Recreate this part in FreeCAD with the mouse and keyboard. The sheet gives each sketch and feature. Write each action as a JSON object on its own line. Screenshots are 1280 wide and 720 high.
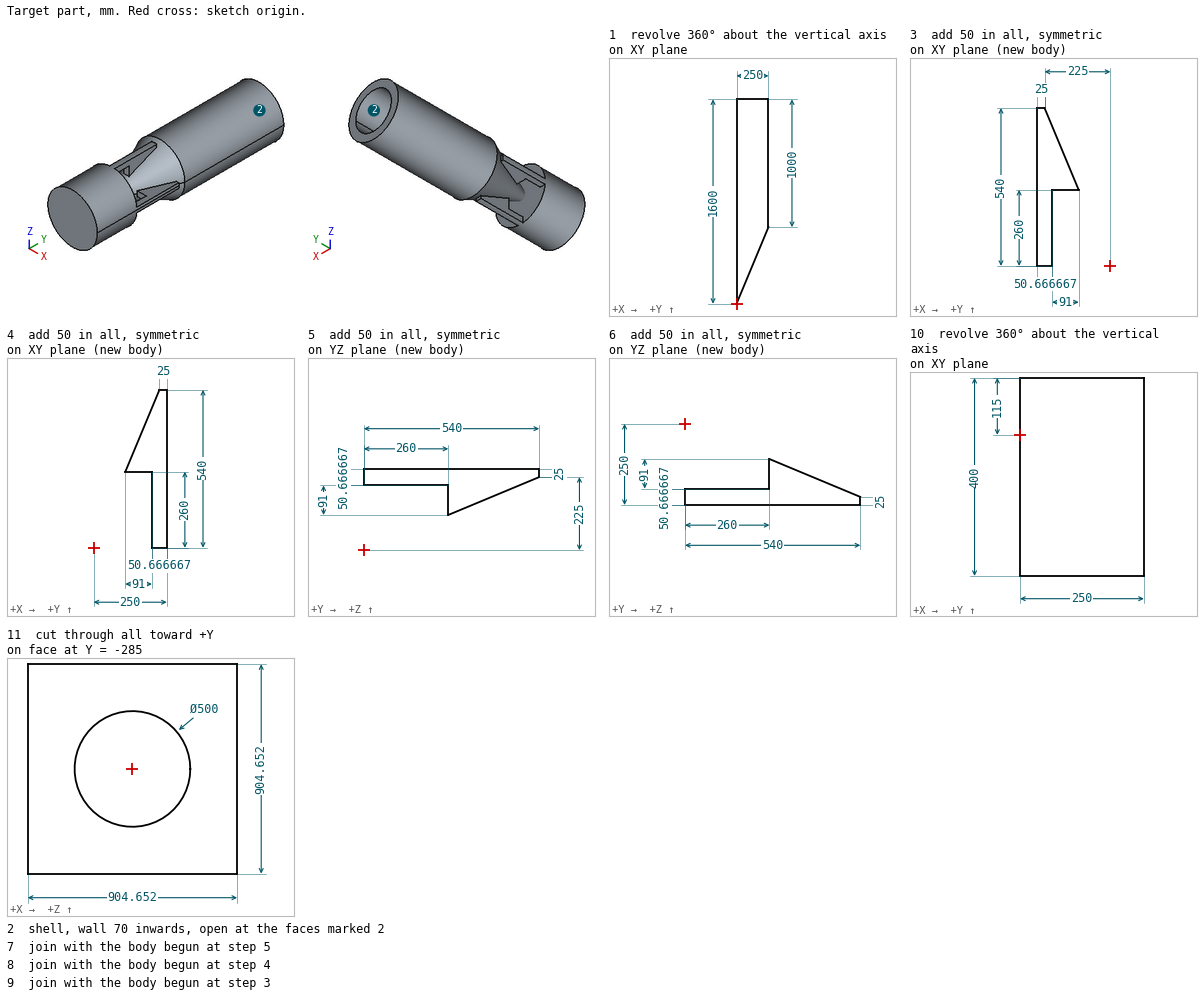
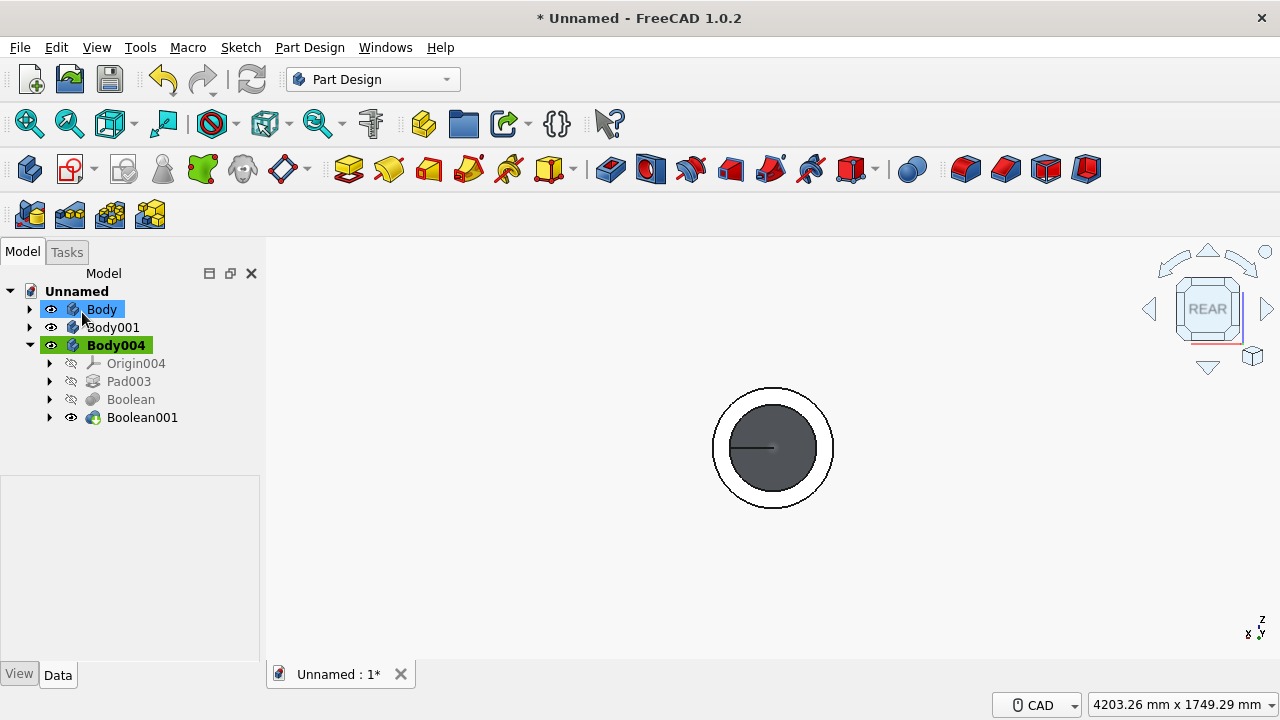
{"action": "left_click", "coordinate": [30, 124]}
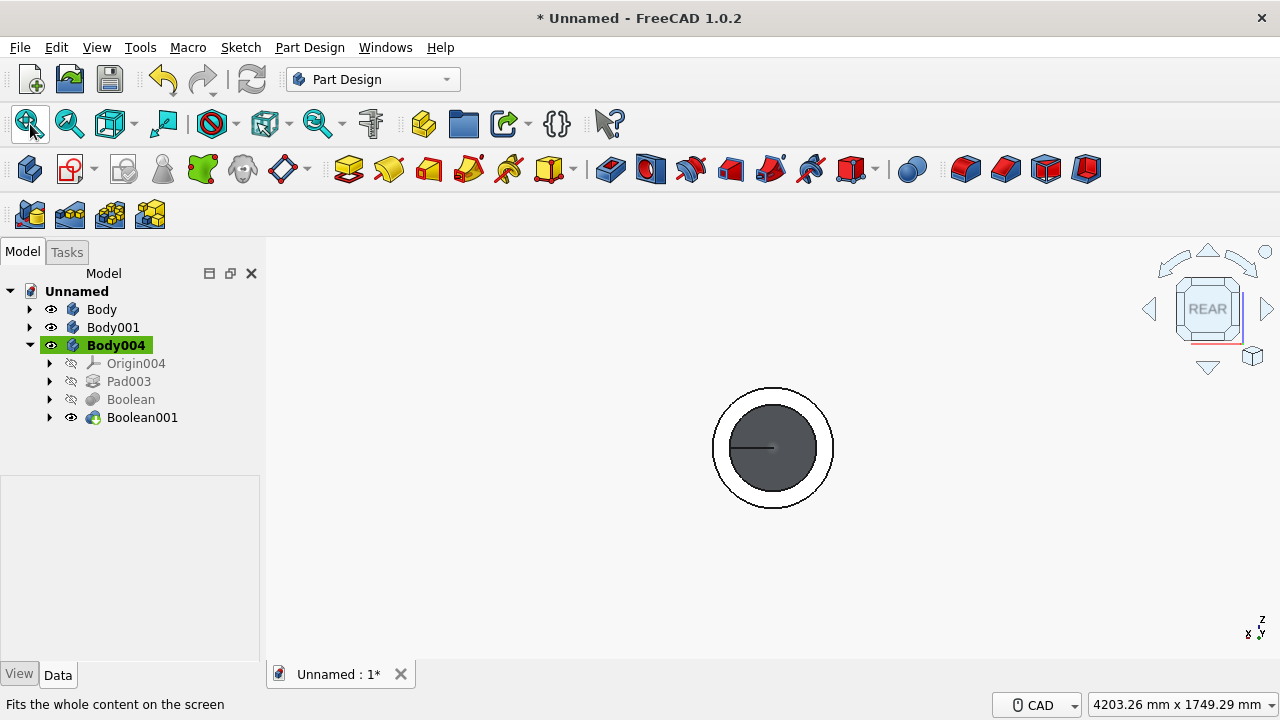
{"action": "left_click", "coordinate": [96, 327]}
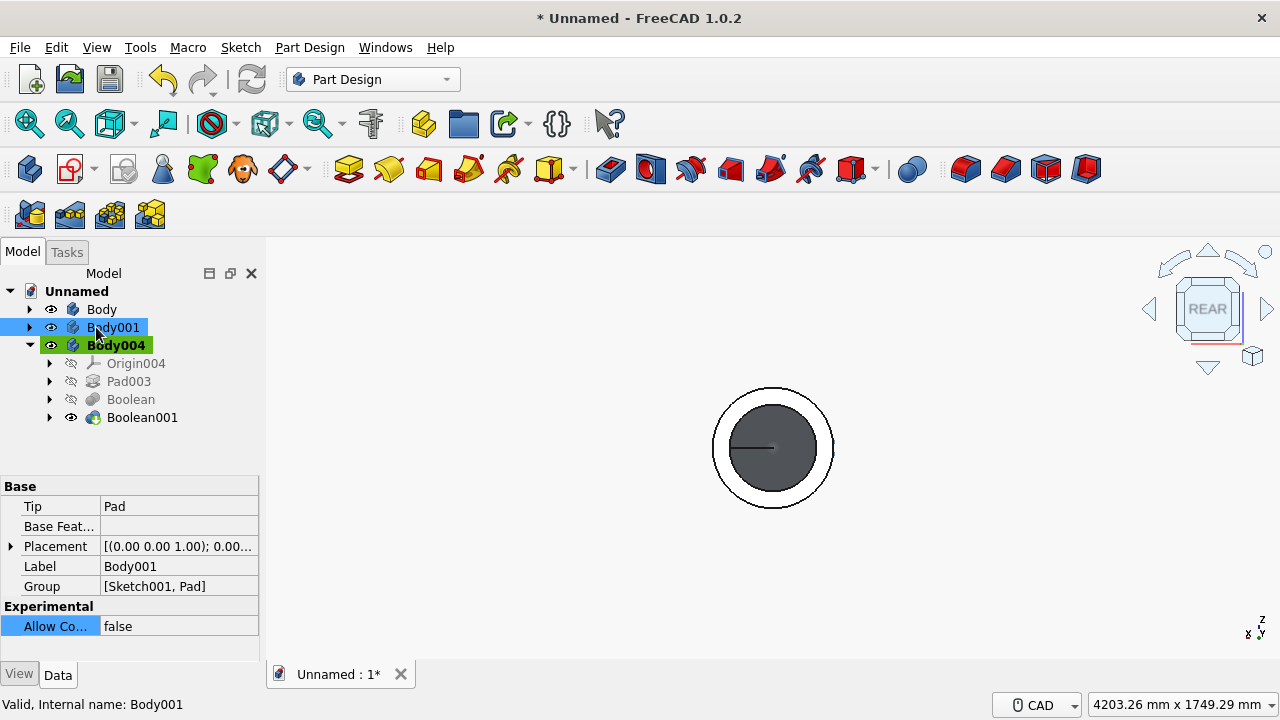
{"action": "left_click", "coordinate": [914, 170]}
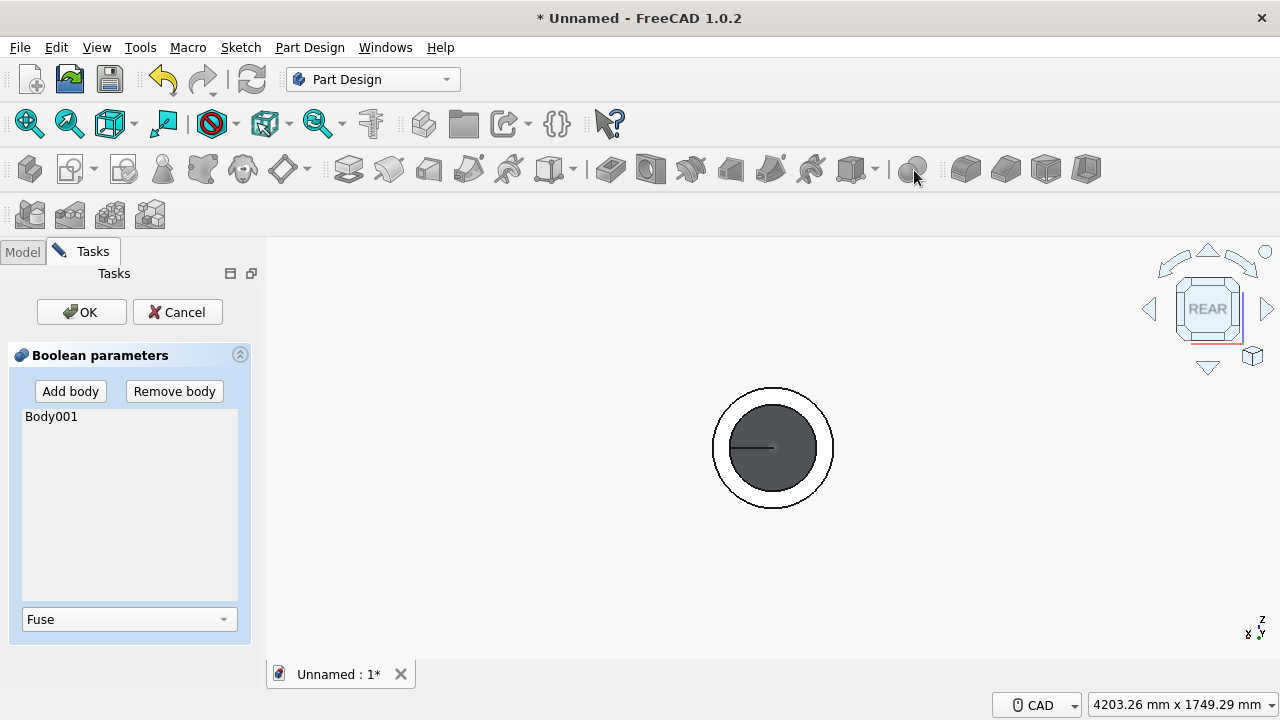
{"action": "left_click", "coordinate": [82, 312]}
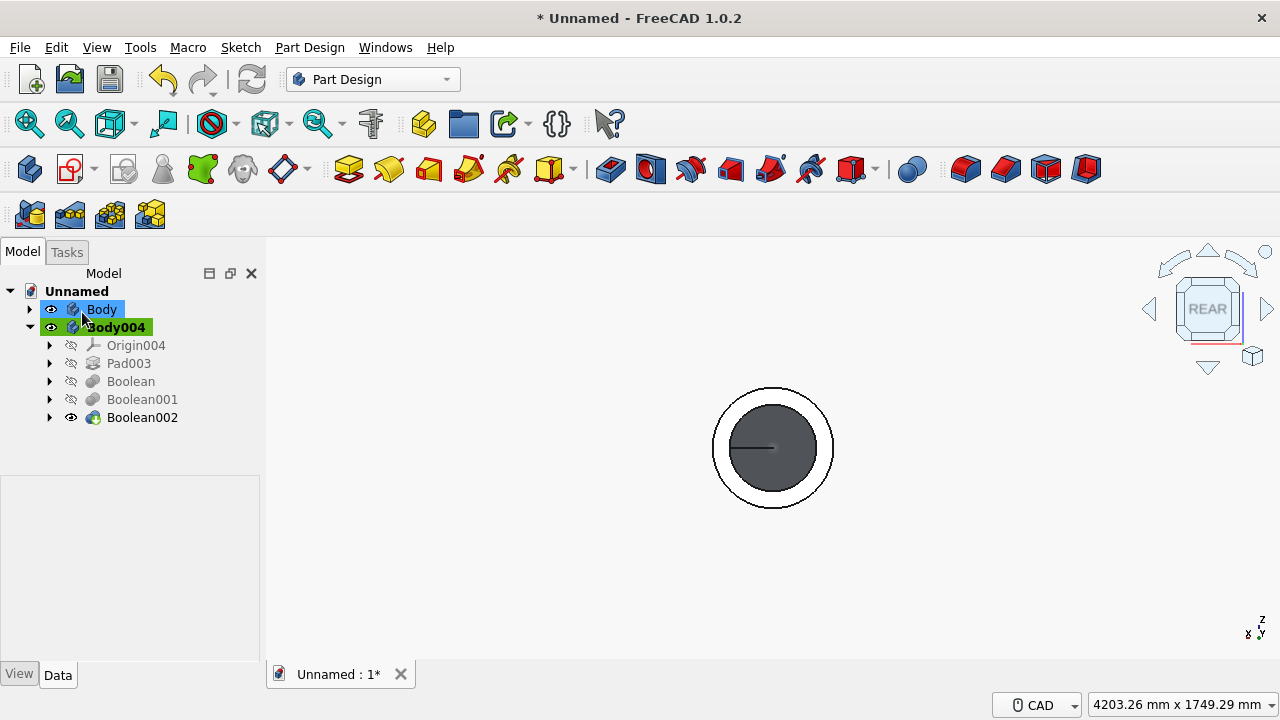
{"action": "left_click", "coordinate": [30, 124]}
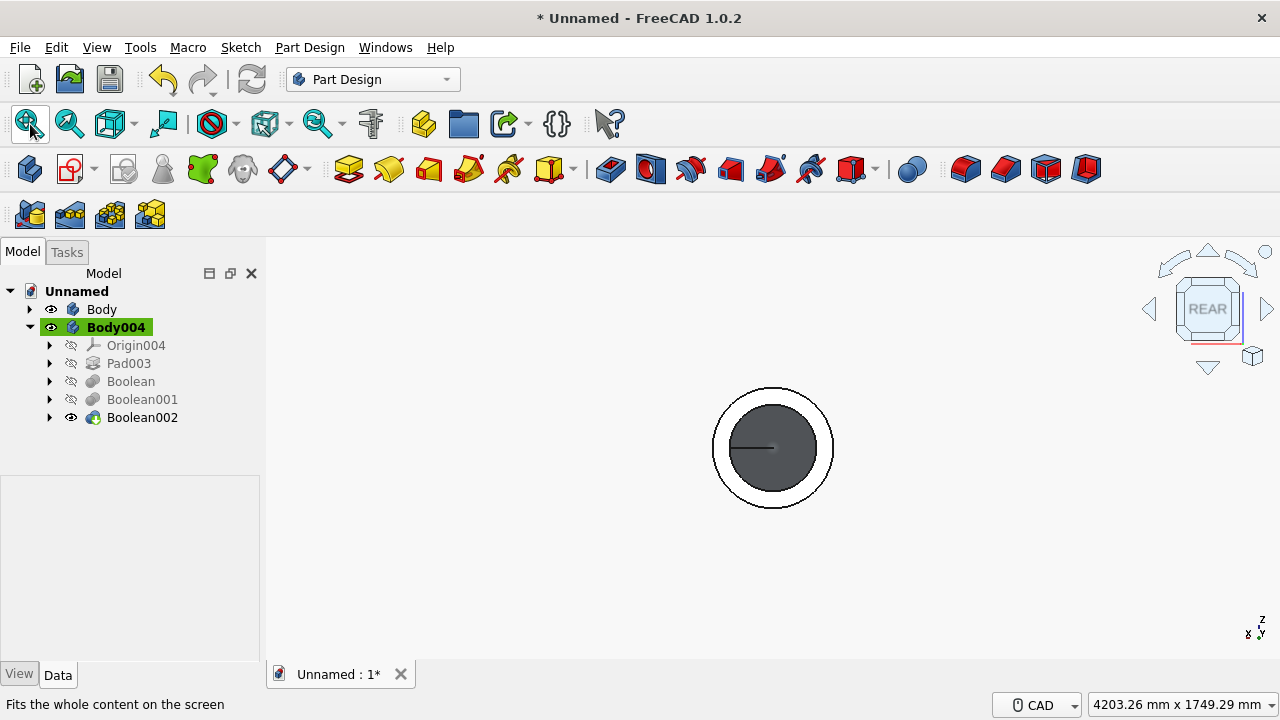
{"action": "left_click", "coordinate": [70, 170]}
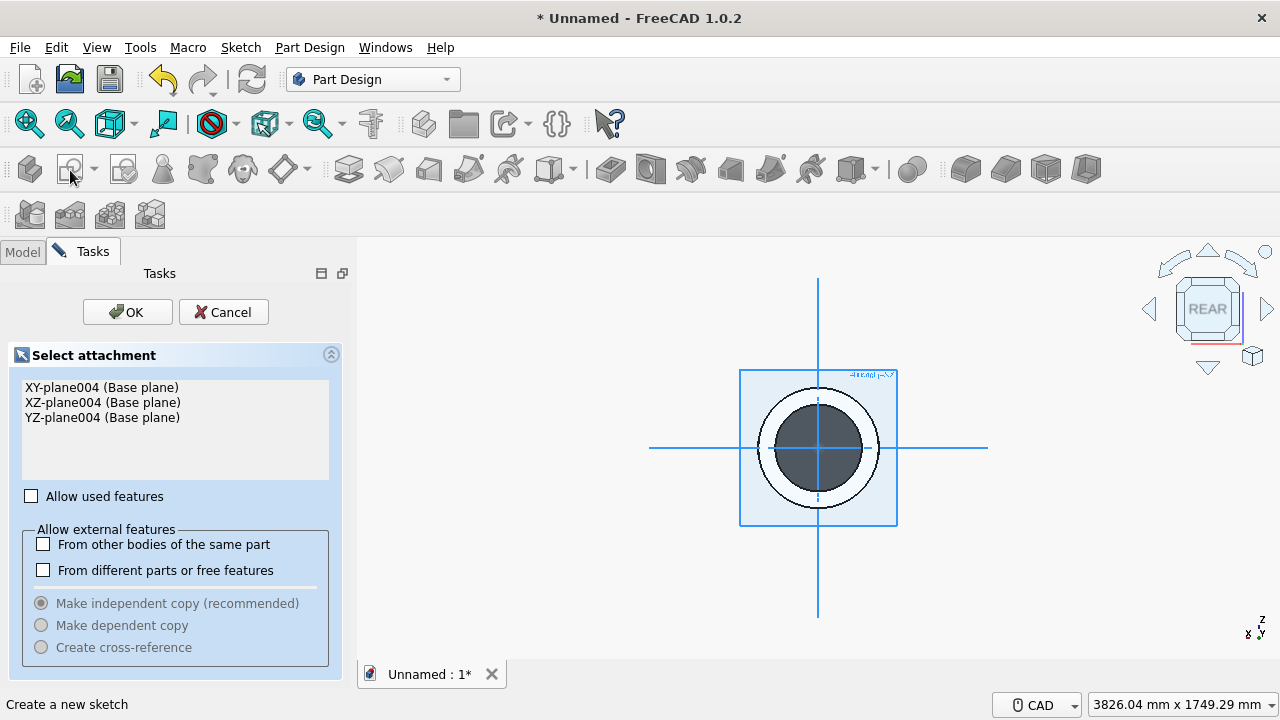
{"action": "left_click", "coordinate": [82, 388]}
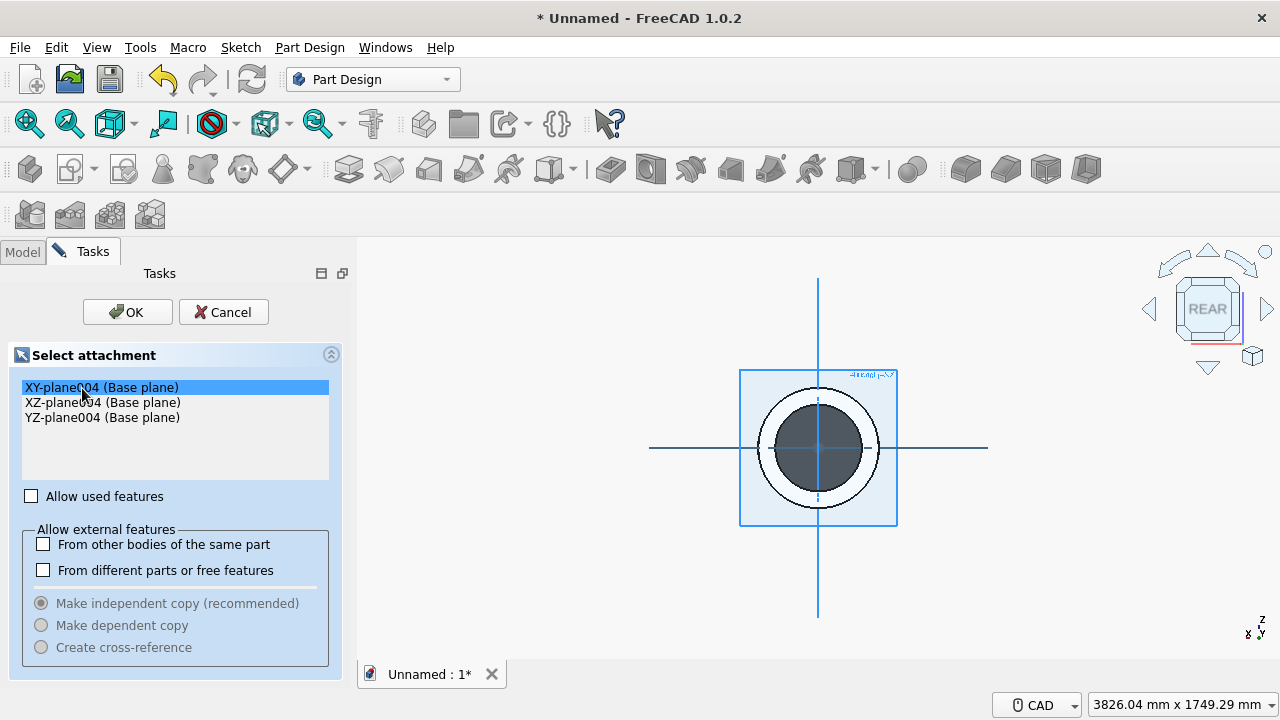
{"action": "left_click", "coordinate": [128, 312]}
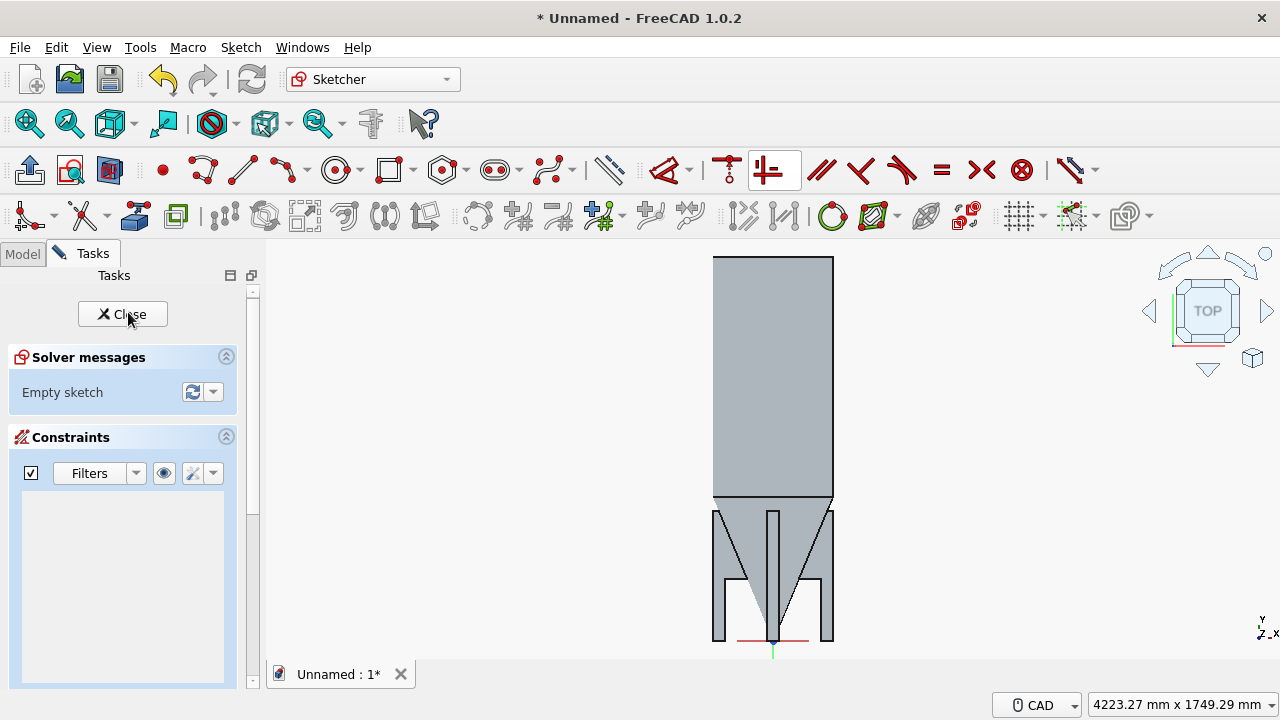
{"action": "left_click", "coordinate": [110, 170]}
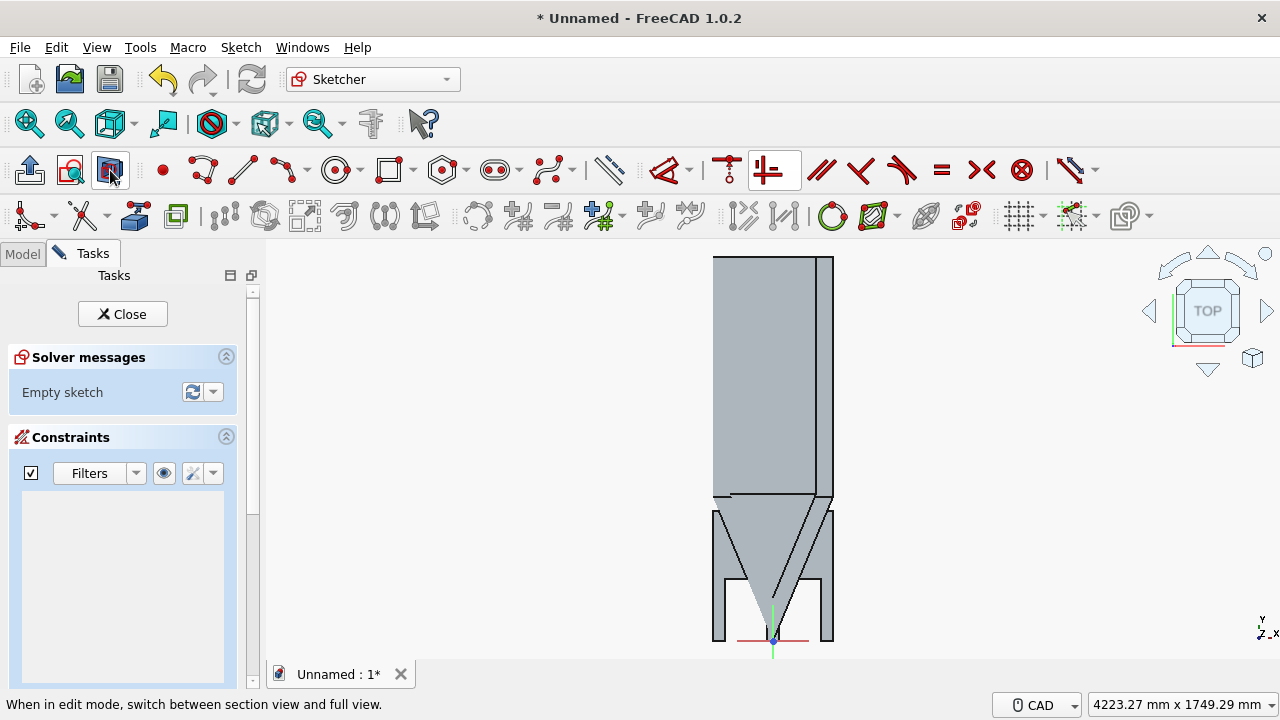
{"action": "scroll", "coordinate": [704, 449], "scroll_direction": "down", "scroll_amount": 5}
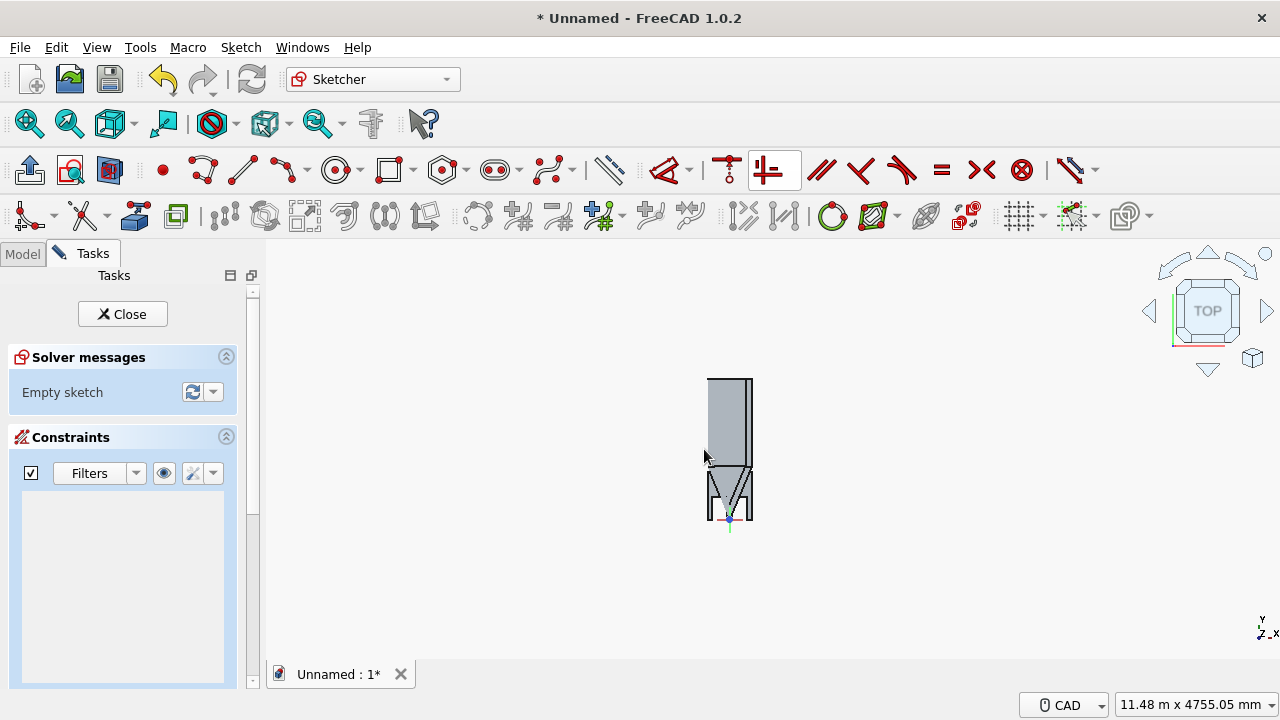
{"action": "scroll", "coordinate": [746, 540], "scroll_direction": "up", "scroll_amount": 10}